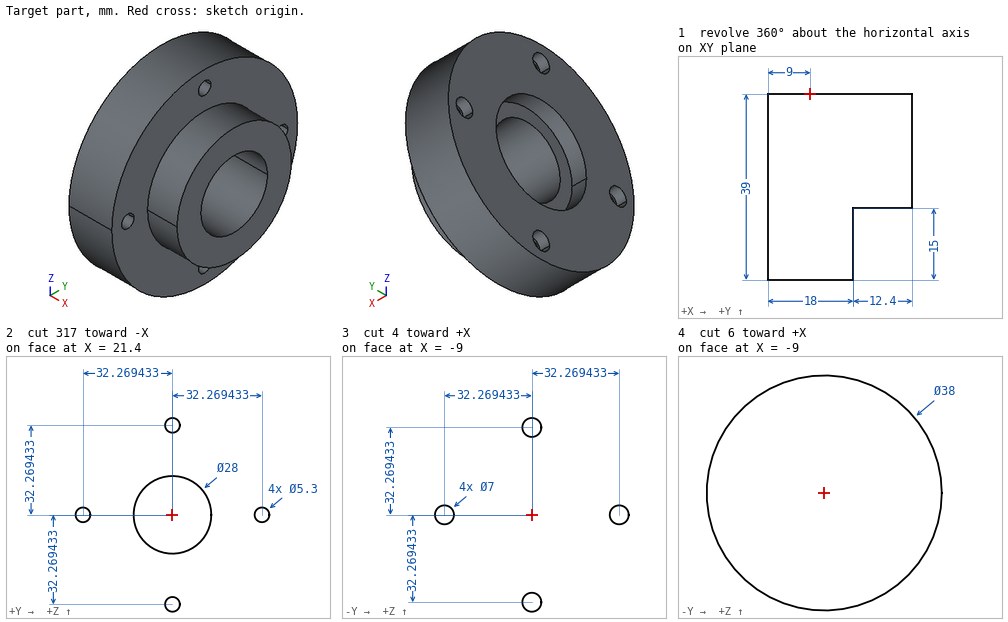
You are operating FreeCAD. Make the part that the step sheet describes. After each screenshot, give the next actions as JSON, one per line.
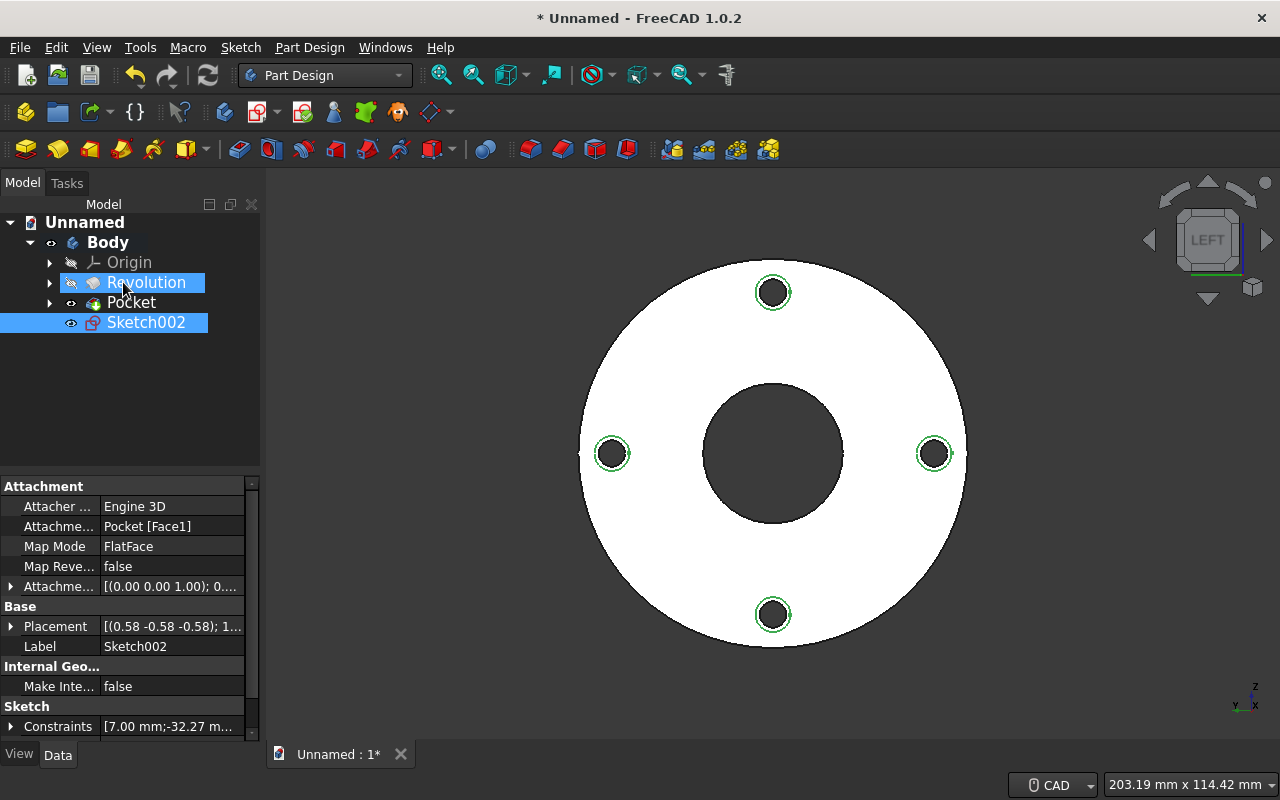
{"action": "left_click", "coordinate": [240, 150]}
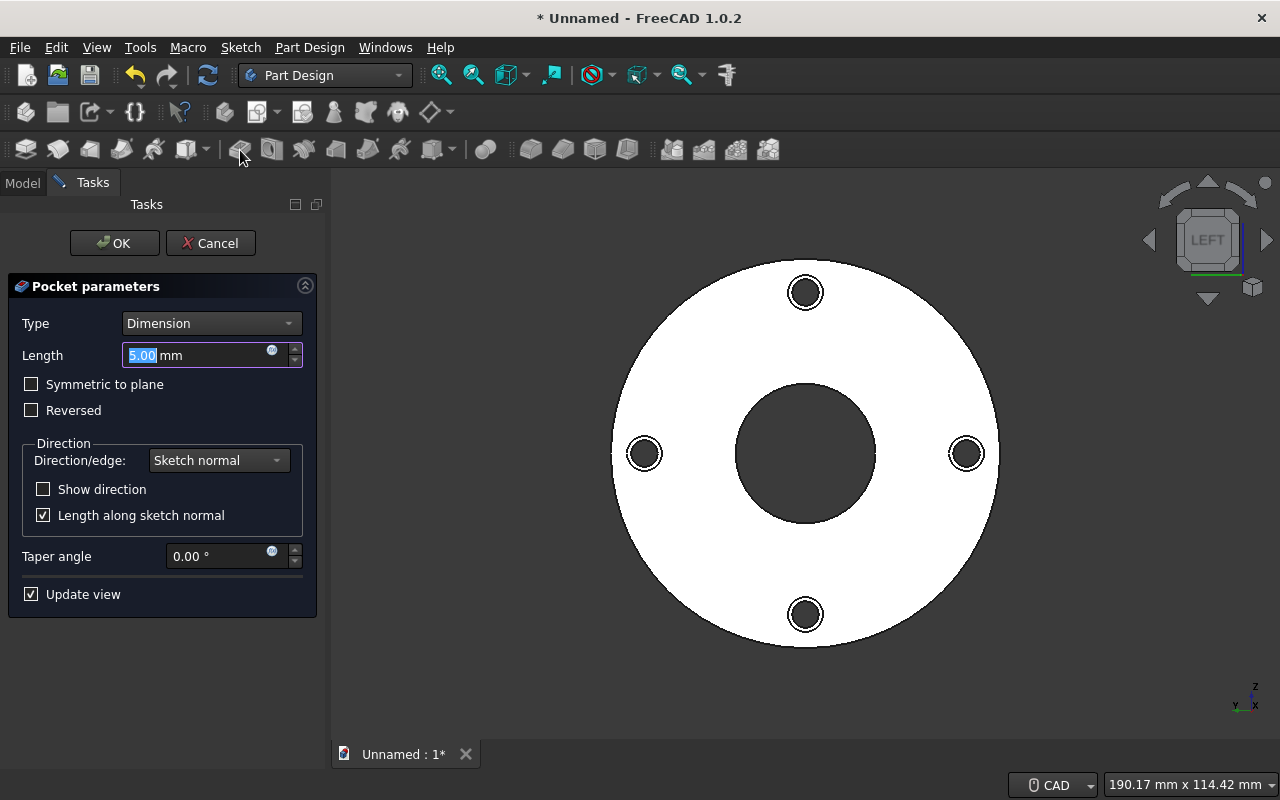
{"action": "type", "text": "4"}
{"action": "key", "text": "Tab"}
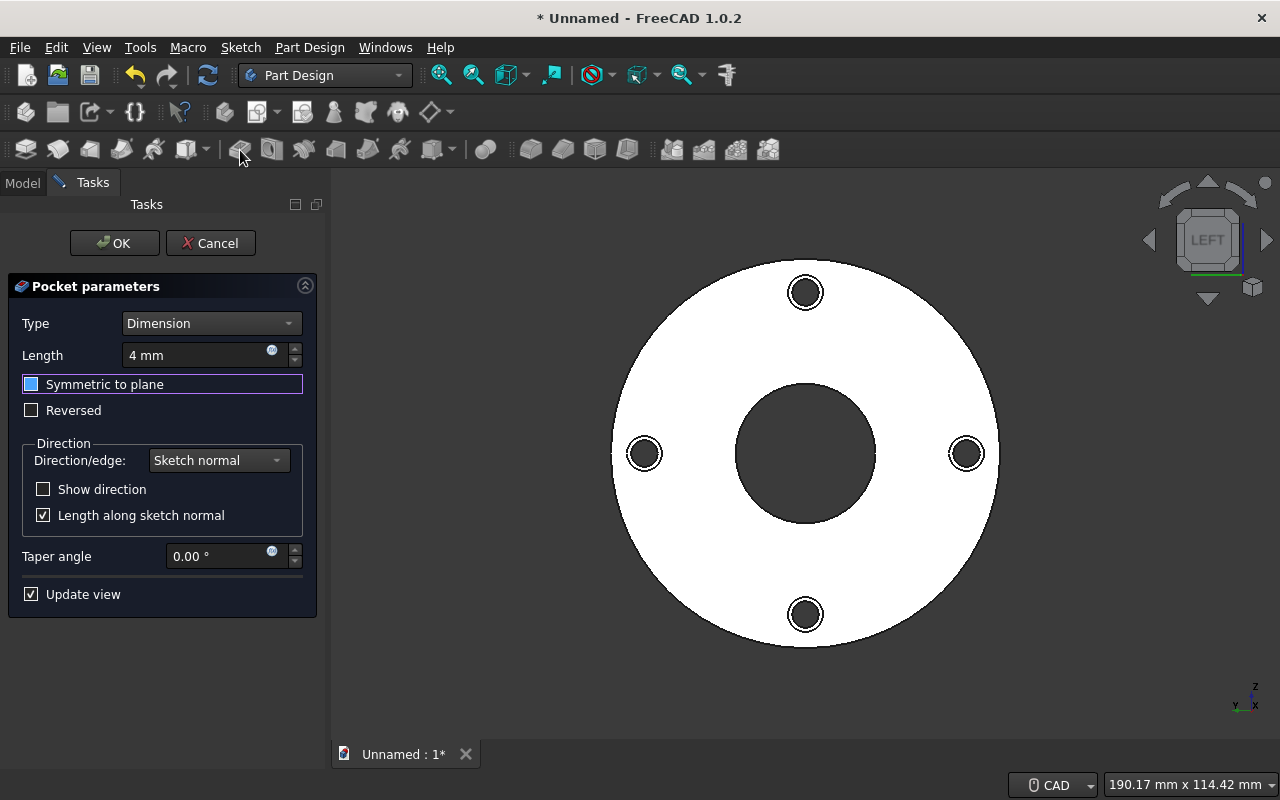
{"action": "left_click", "coordinate": [115, 243]}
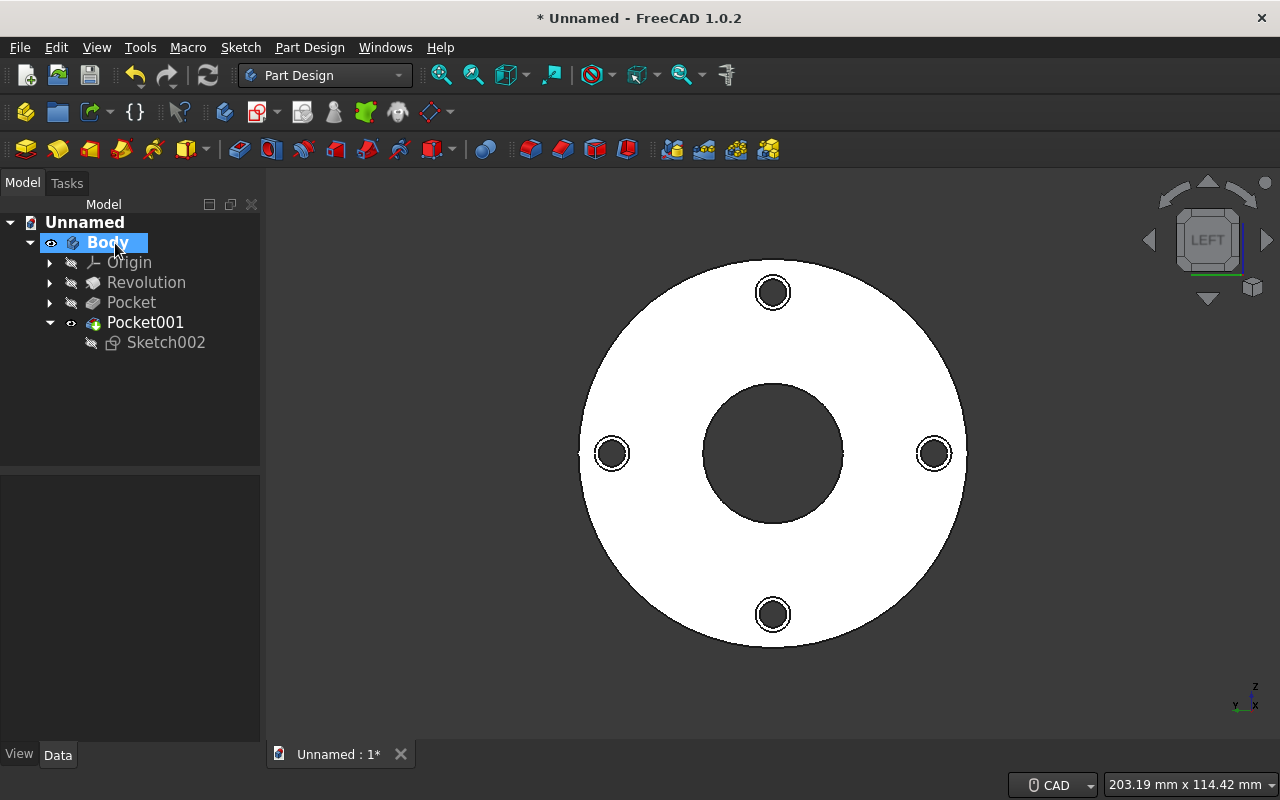
{"action": "left_click", "coordinate": [662, 397]}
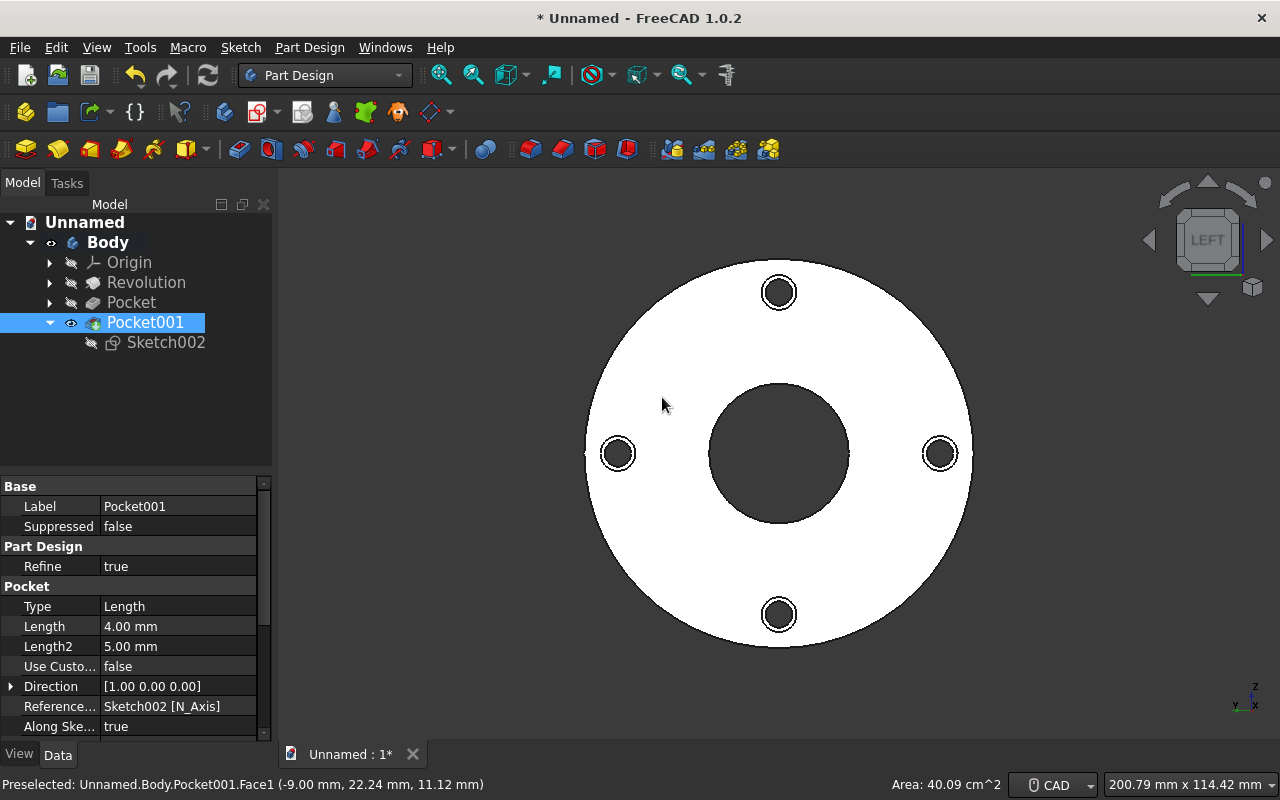
{"action": "left_click", "coordinate": [258, 112]}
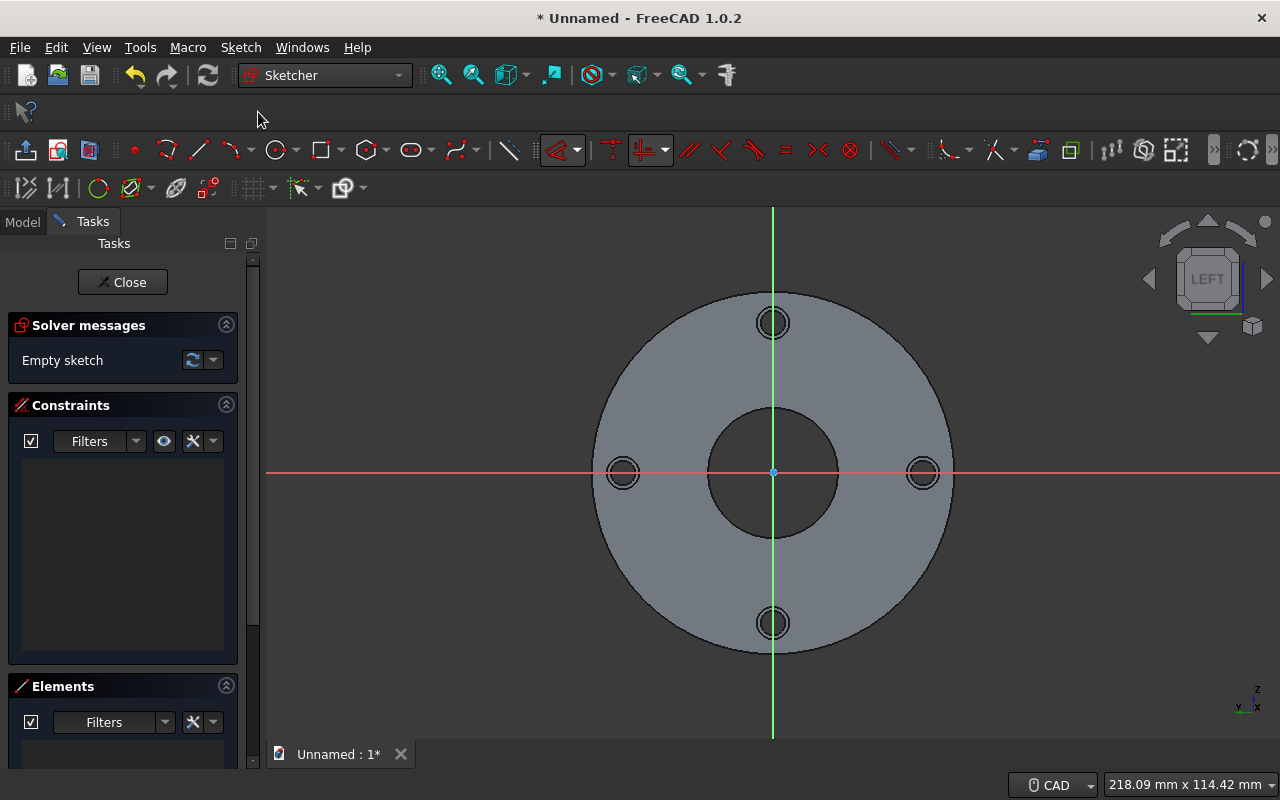
{"action": "scroll", "coordinate": [856, 473], "scroll_direction": "up", "scroll_amount": 3}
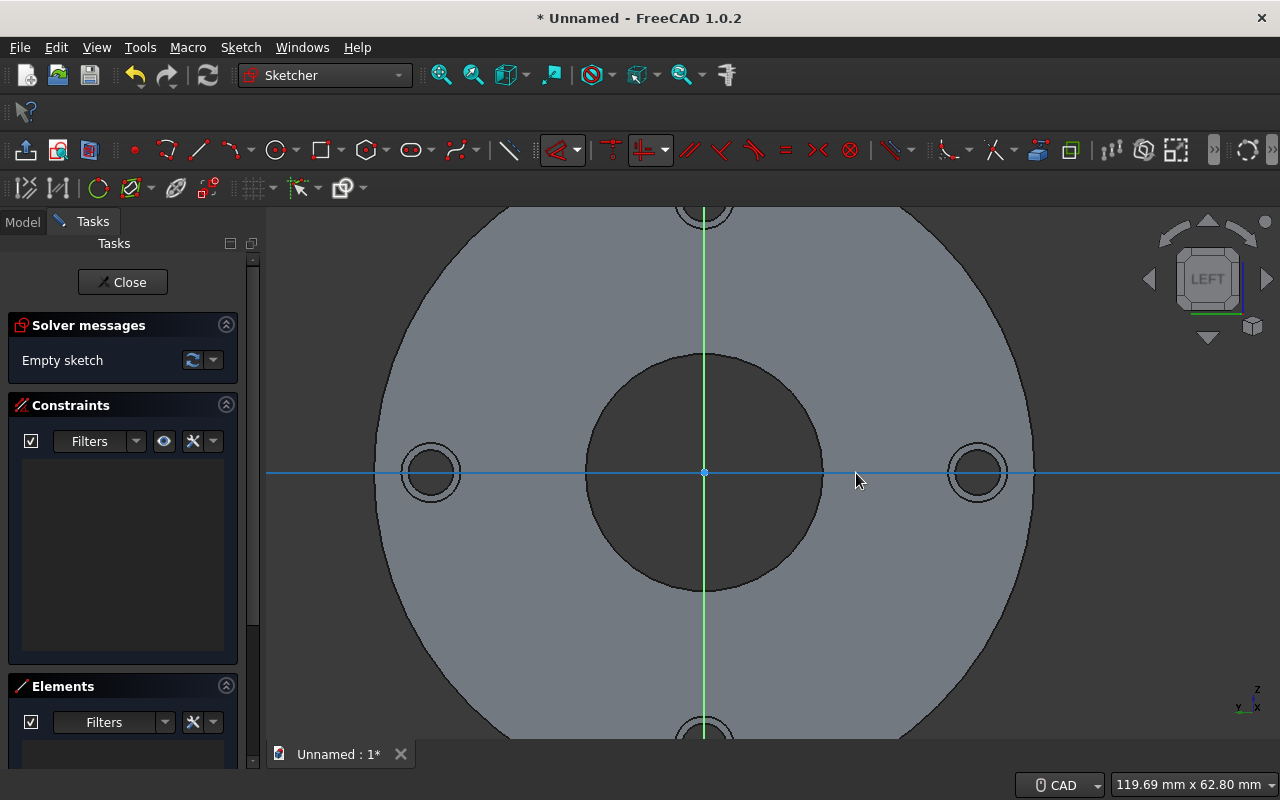
{"action": "left_click", "coordinate": [276, 150]}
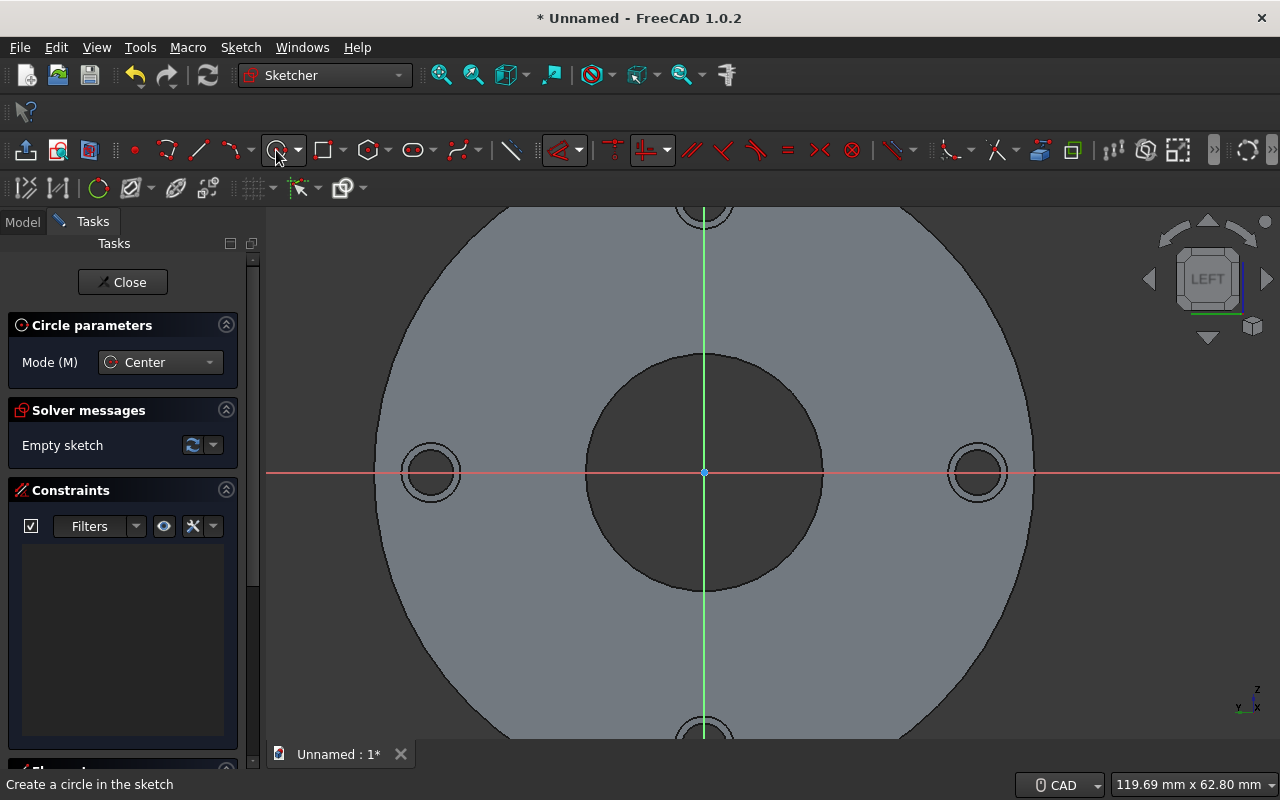
{"action": "left_click", "coordinate": [704, 473]}
{"action": "left_click", "coordinate": [818, 359]}
{"action": "key", "text": "Escape"}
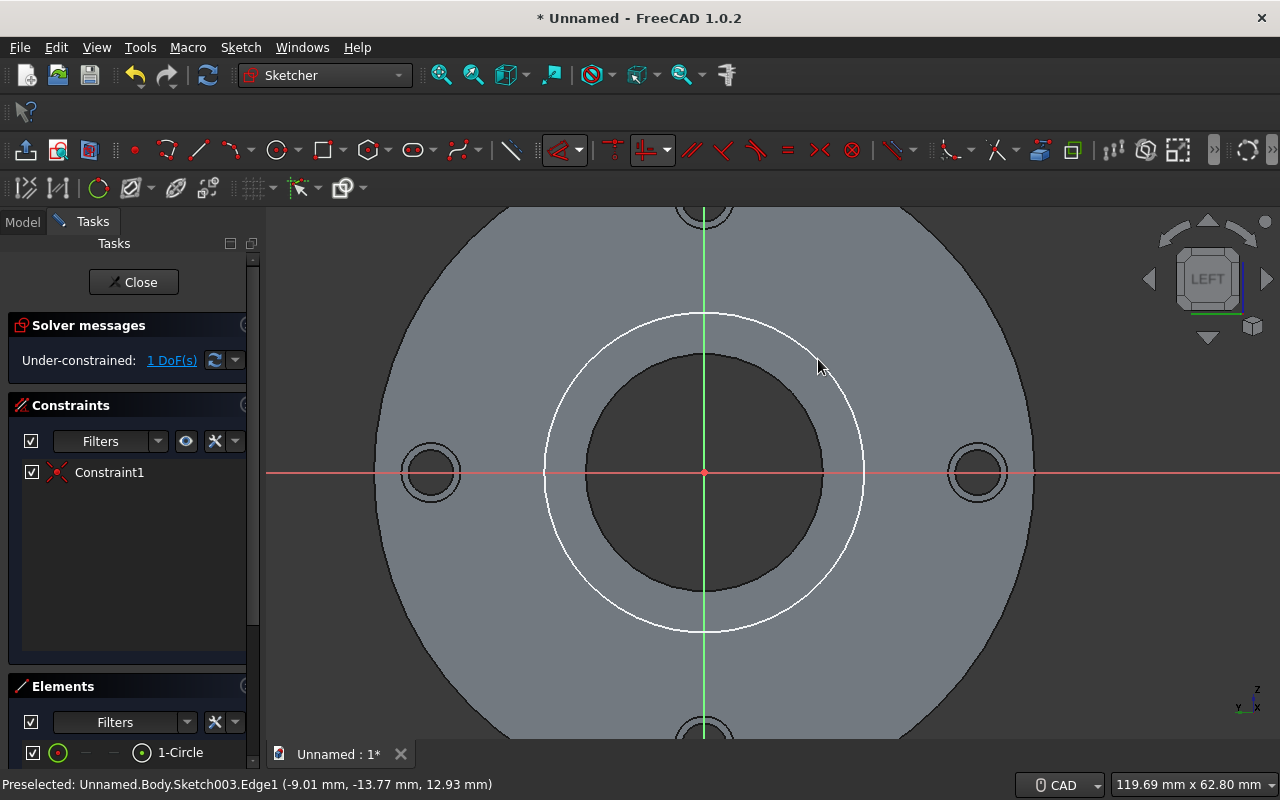
{"action": "left_click", "coordinate": [817, 359]}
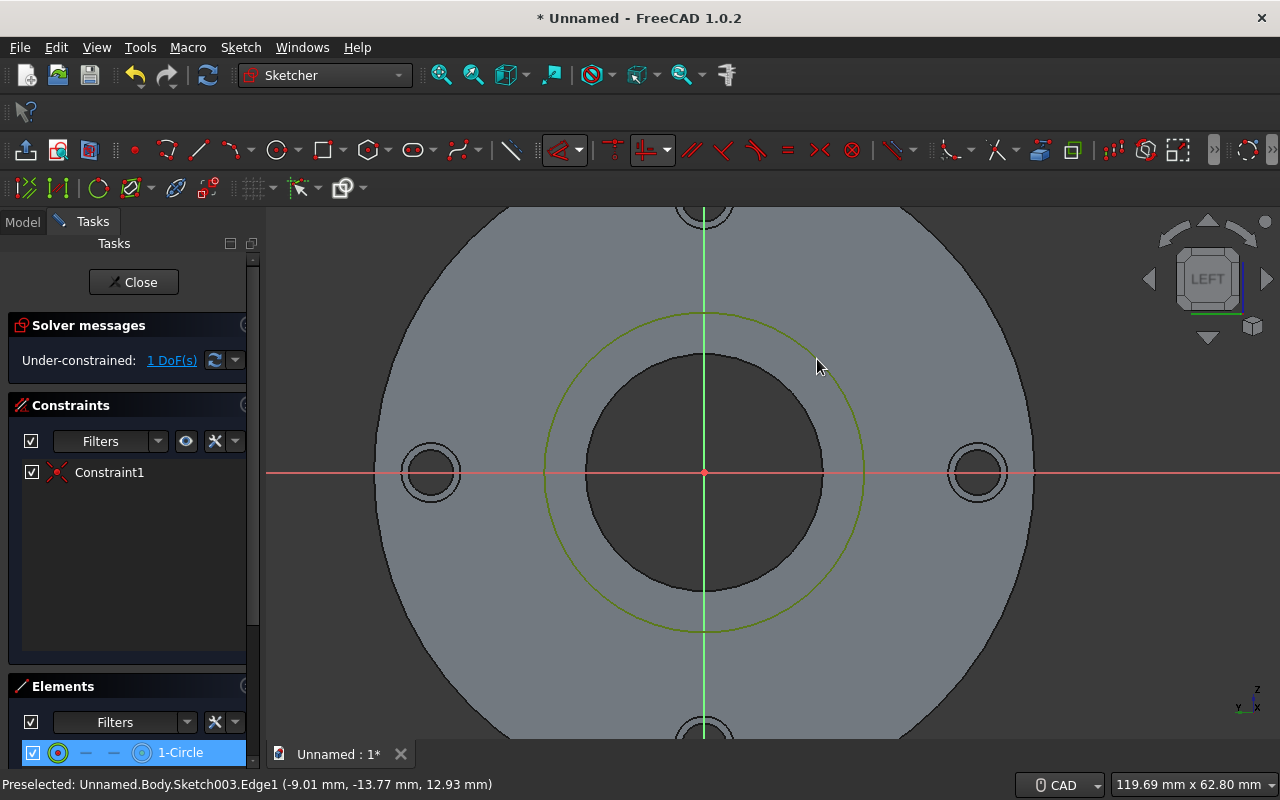
{"action": "key", "text": "k o"}